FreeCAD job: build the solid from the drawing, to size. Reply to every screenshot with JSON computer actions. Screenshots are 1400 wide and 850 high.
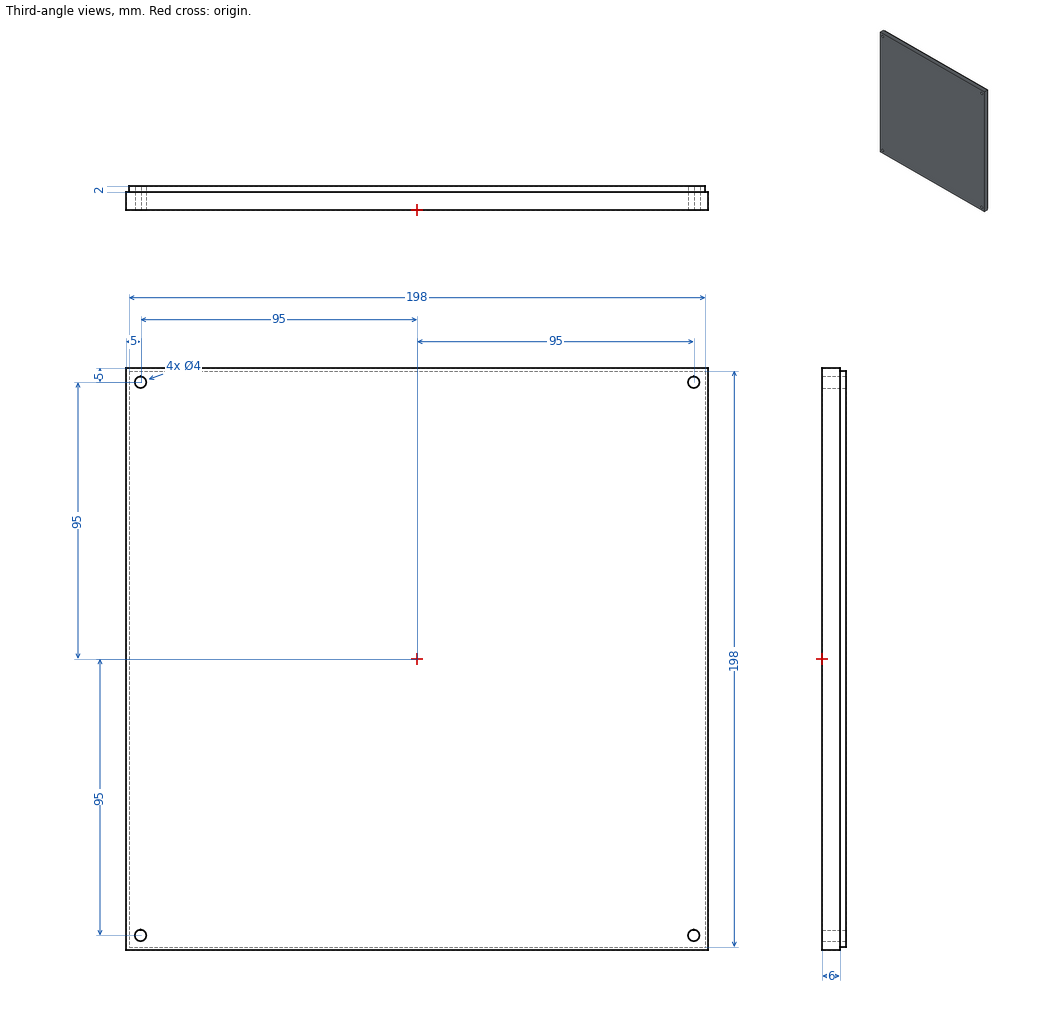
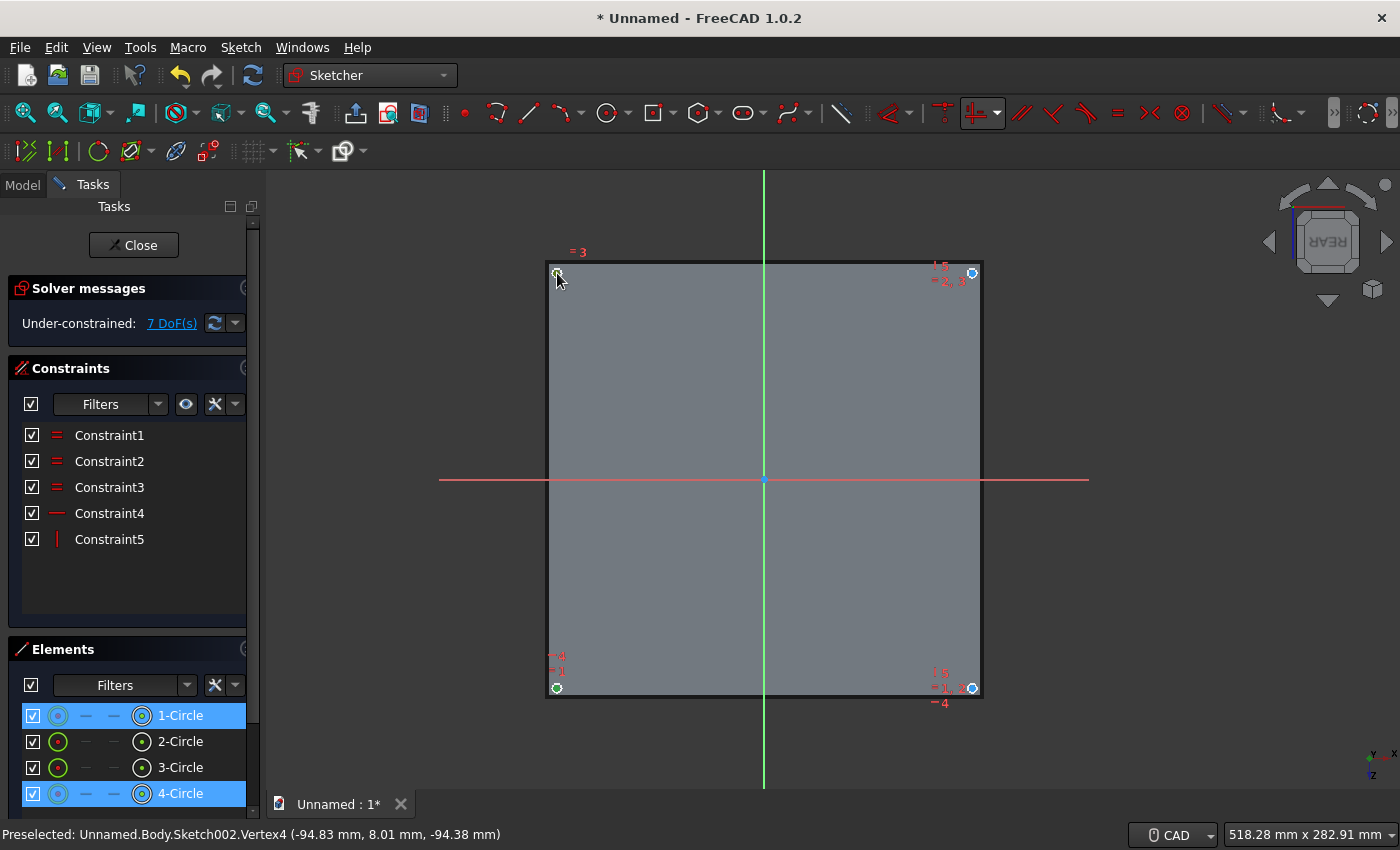
{"action": "left_click", "coordinate": [1000, 114]}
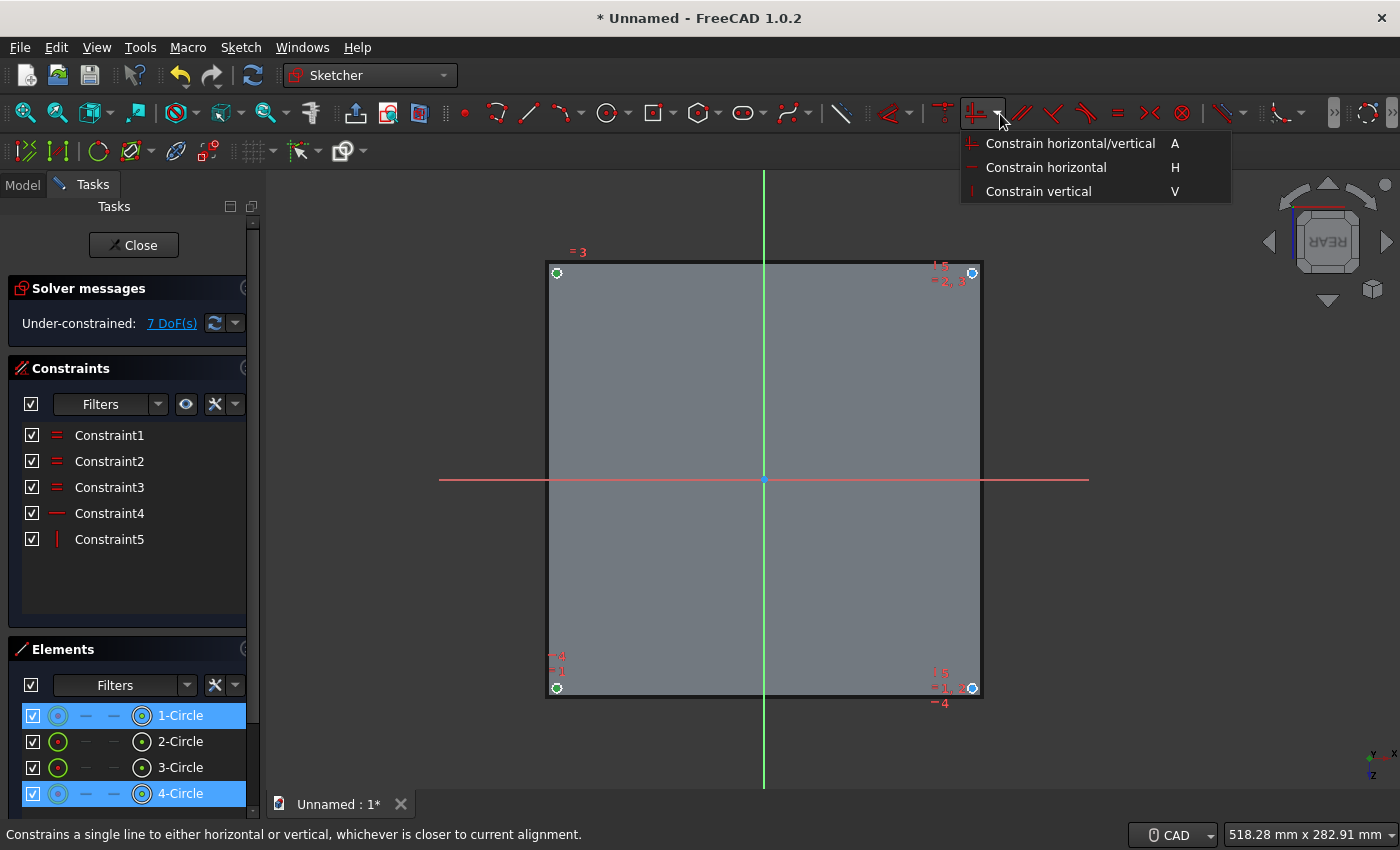
{"action": "left_click", "coordinate": [1096, 191]}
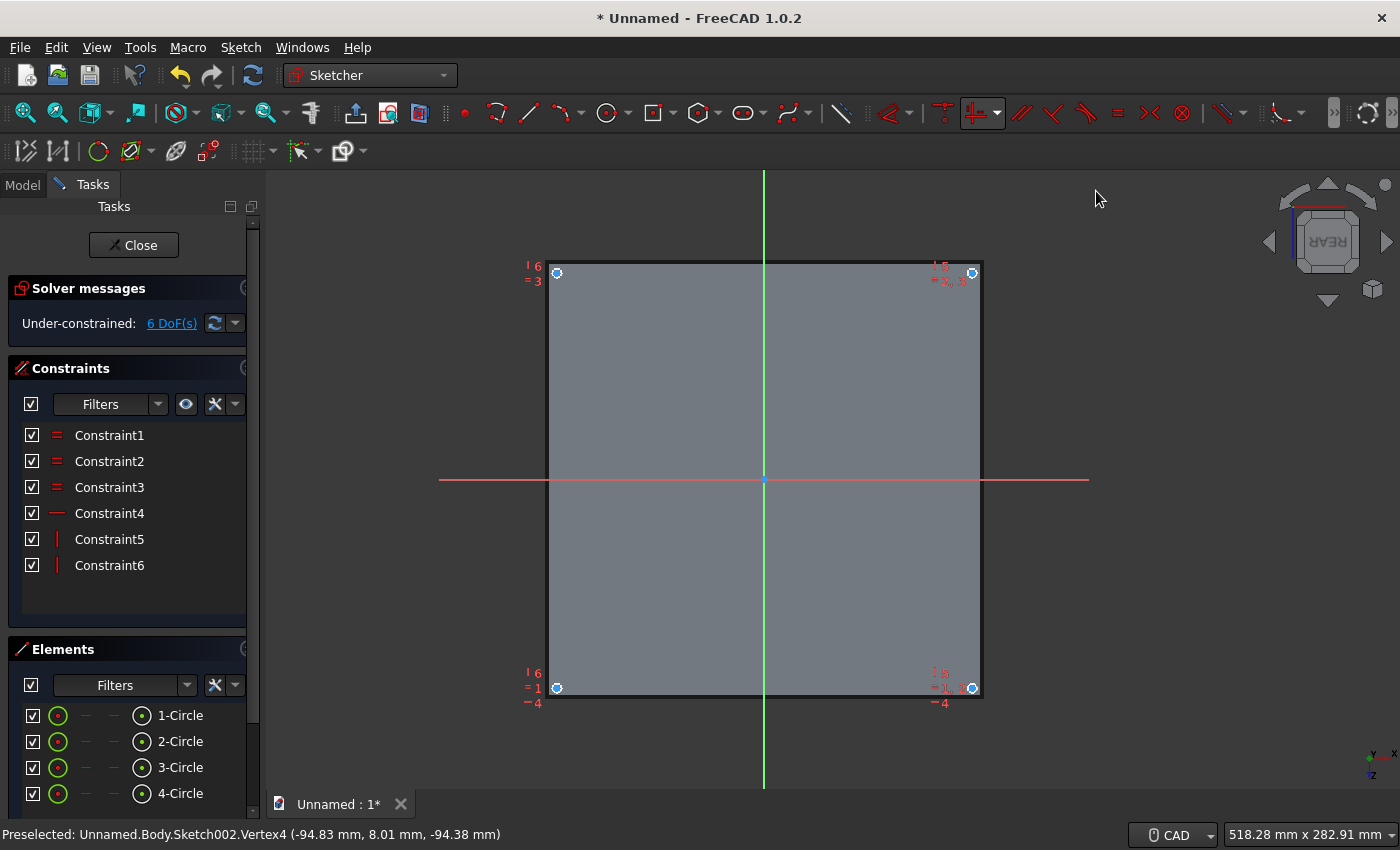
{"action": "left_click", "coordinate": [972, 273]}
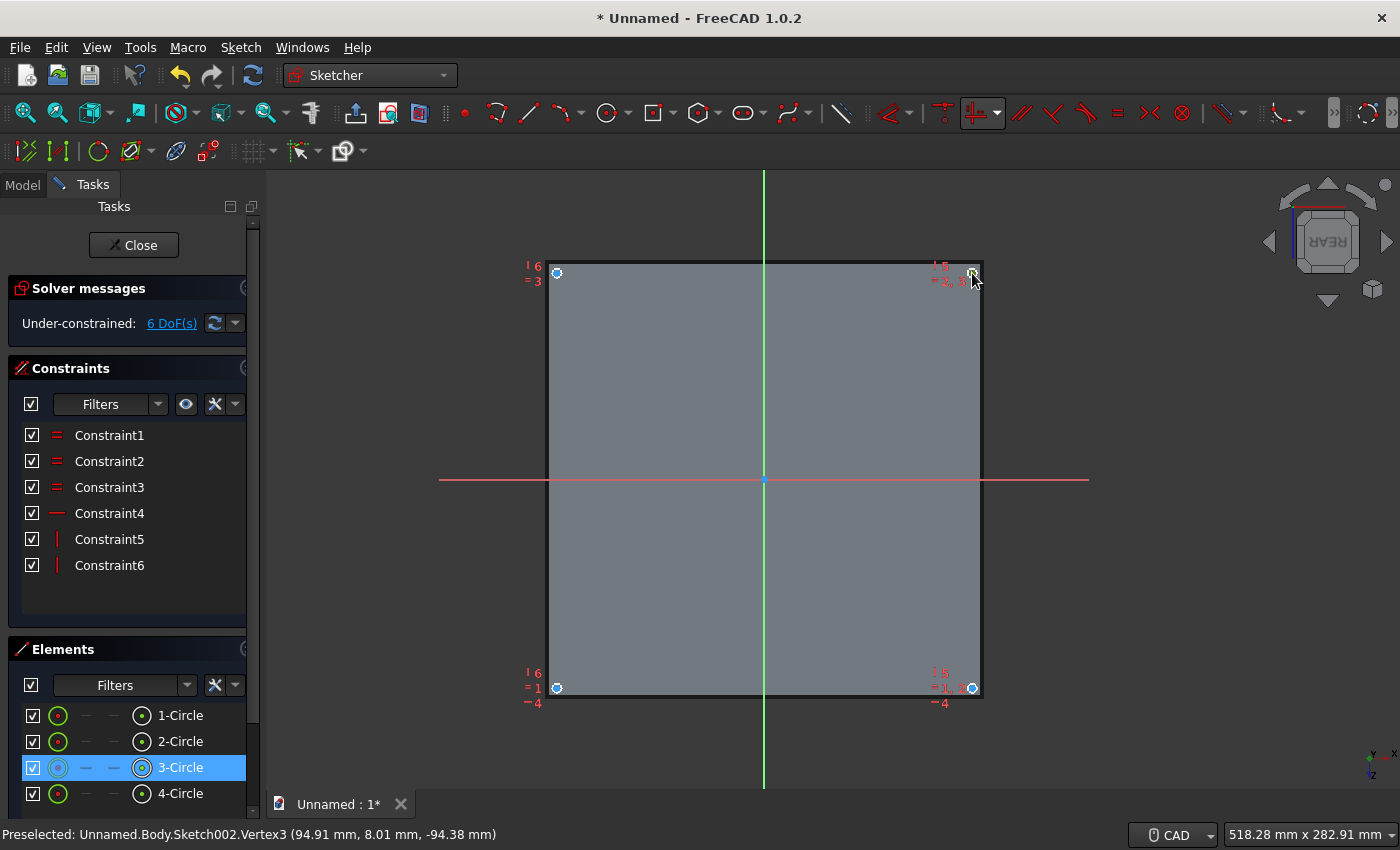
{"action": "left_click", "coordinate": [557, 273]}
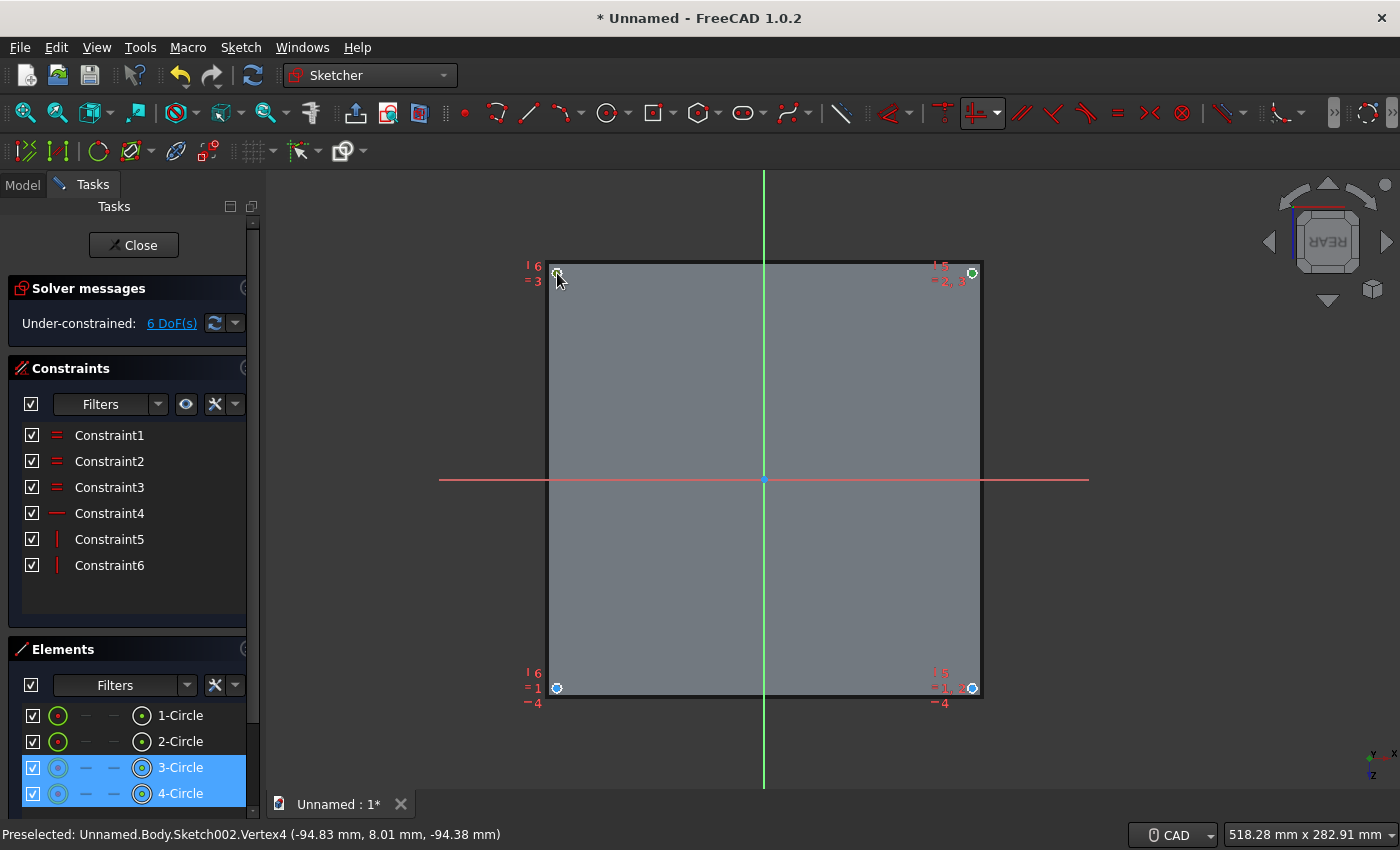
{"action": "key", "text": "h"}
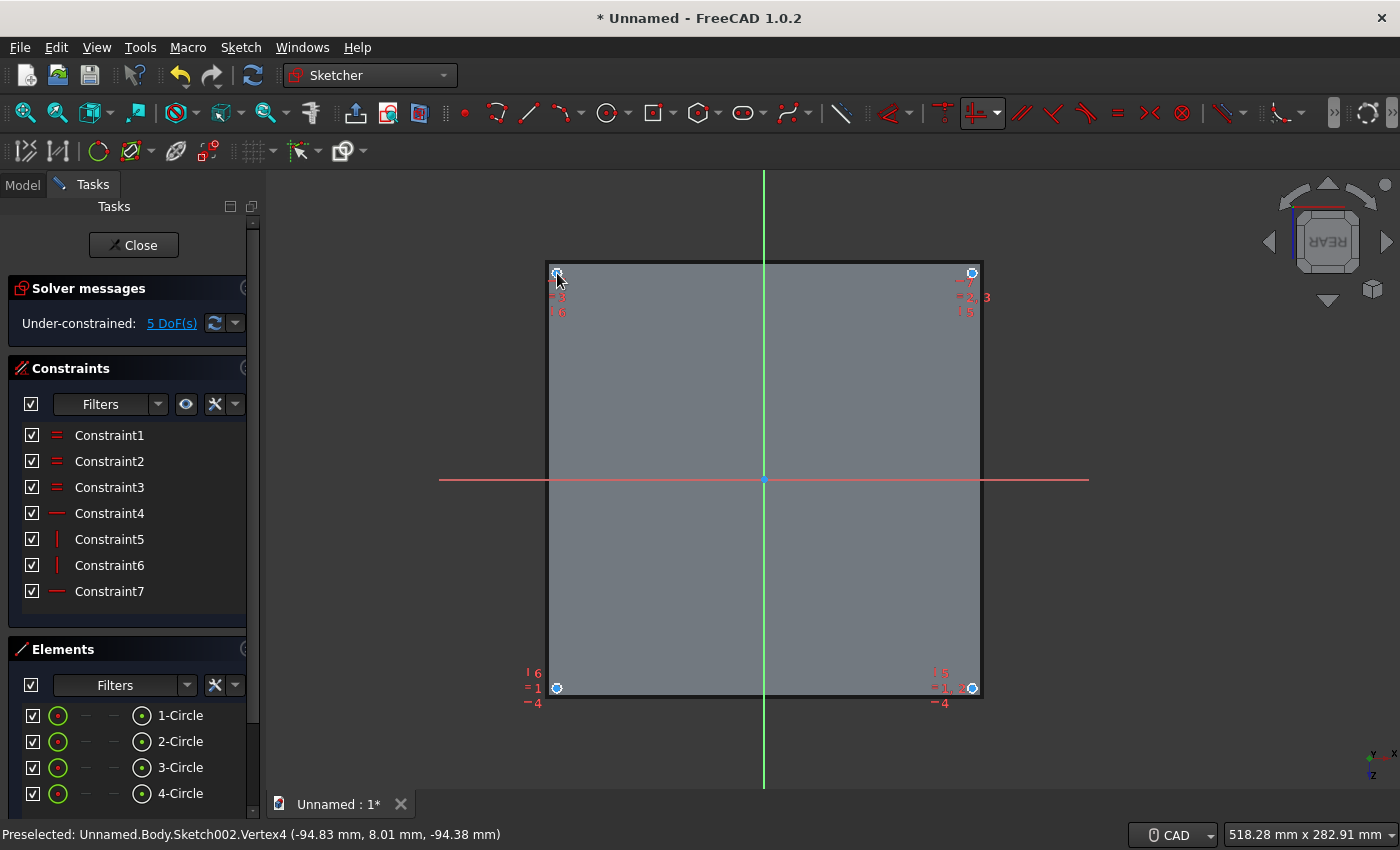
{"action": "left_click", "coordinate": [888, 114]}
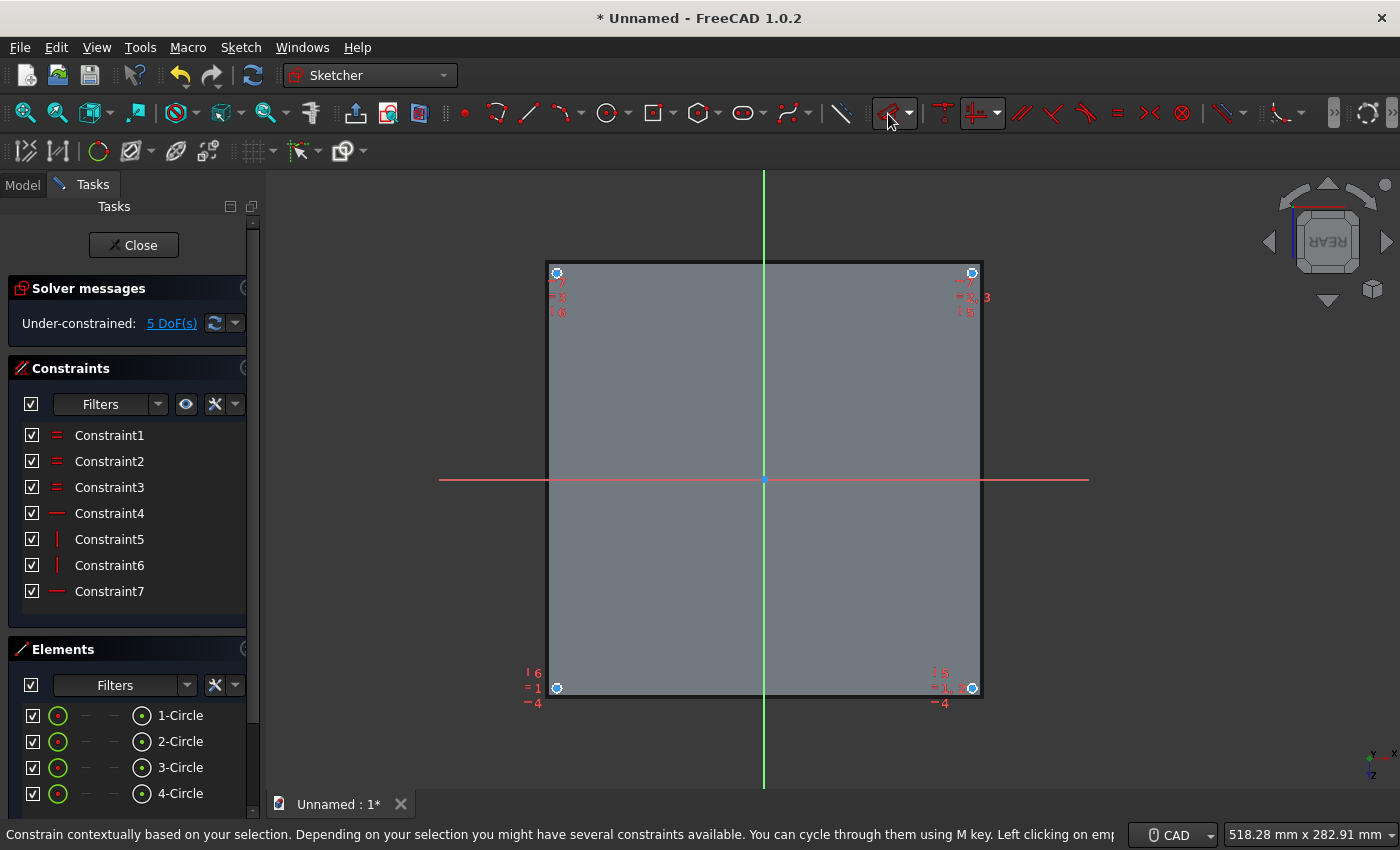
{"action": "scroll", "coordinate": [560, 685], "scroll_direction": "up", "scroll_amount": 8}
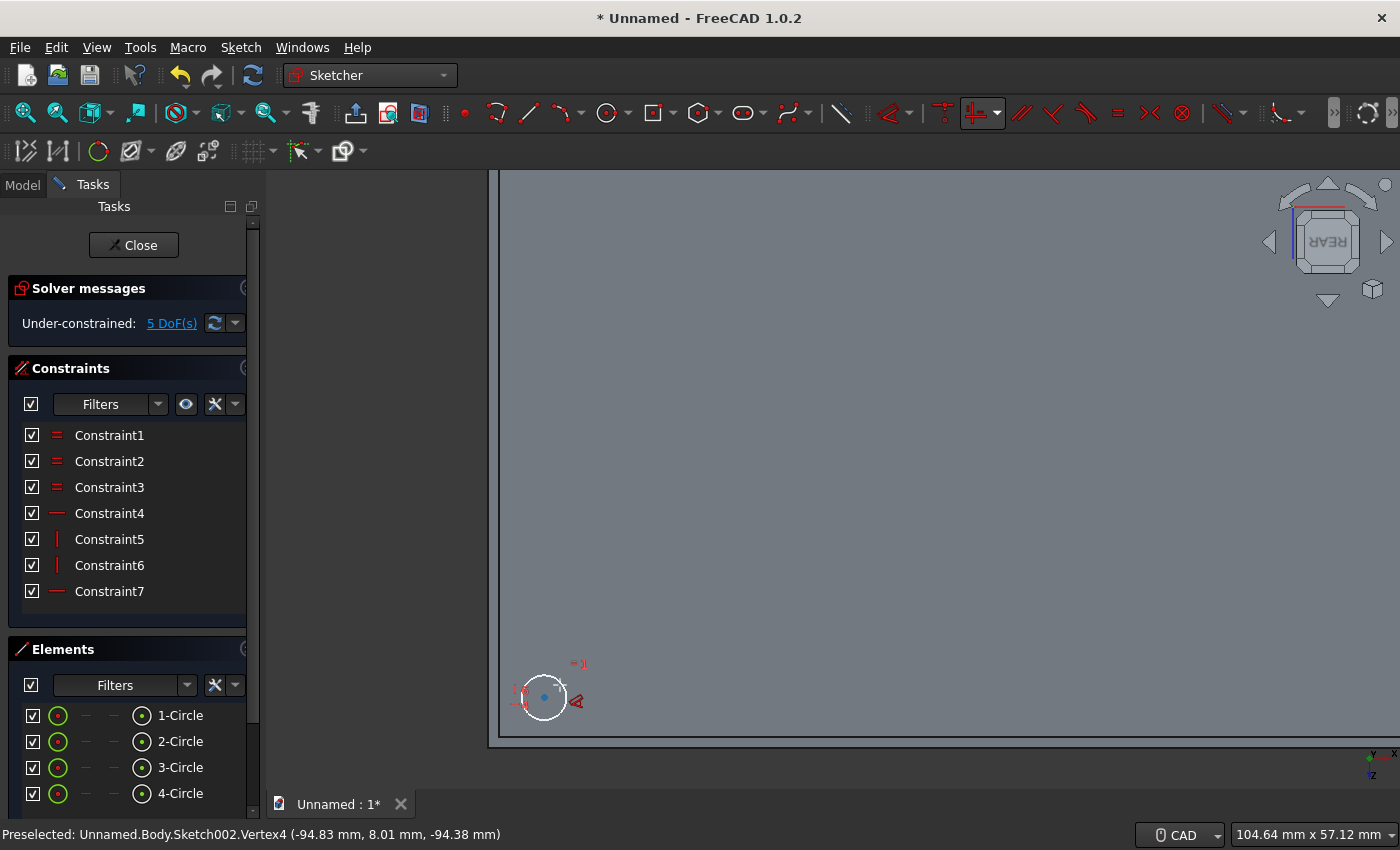
{"action": "left_click", "coordinate": [560, 682]}
{"action": "left_click", "coordinate": [583, 660]}